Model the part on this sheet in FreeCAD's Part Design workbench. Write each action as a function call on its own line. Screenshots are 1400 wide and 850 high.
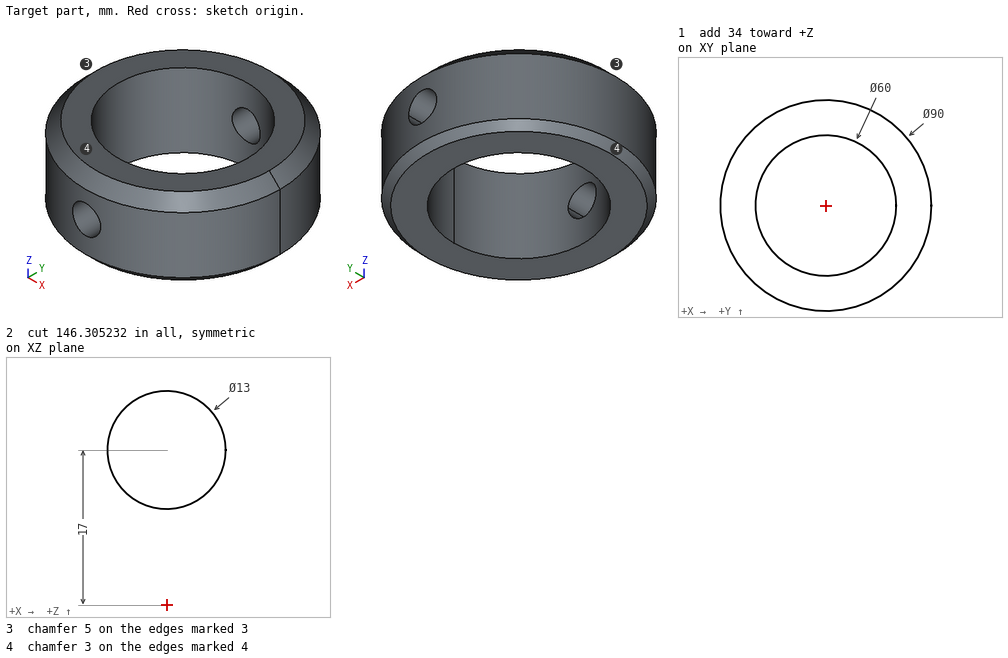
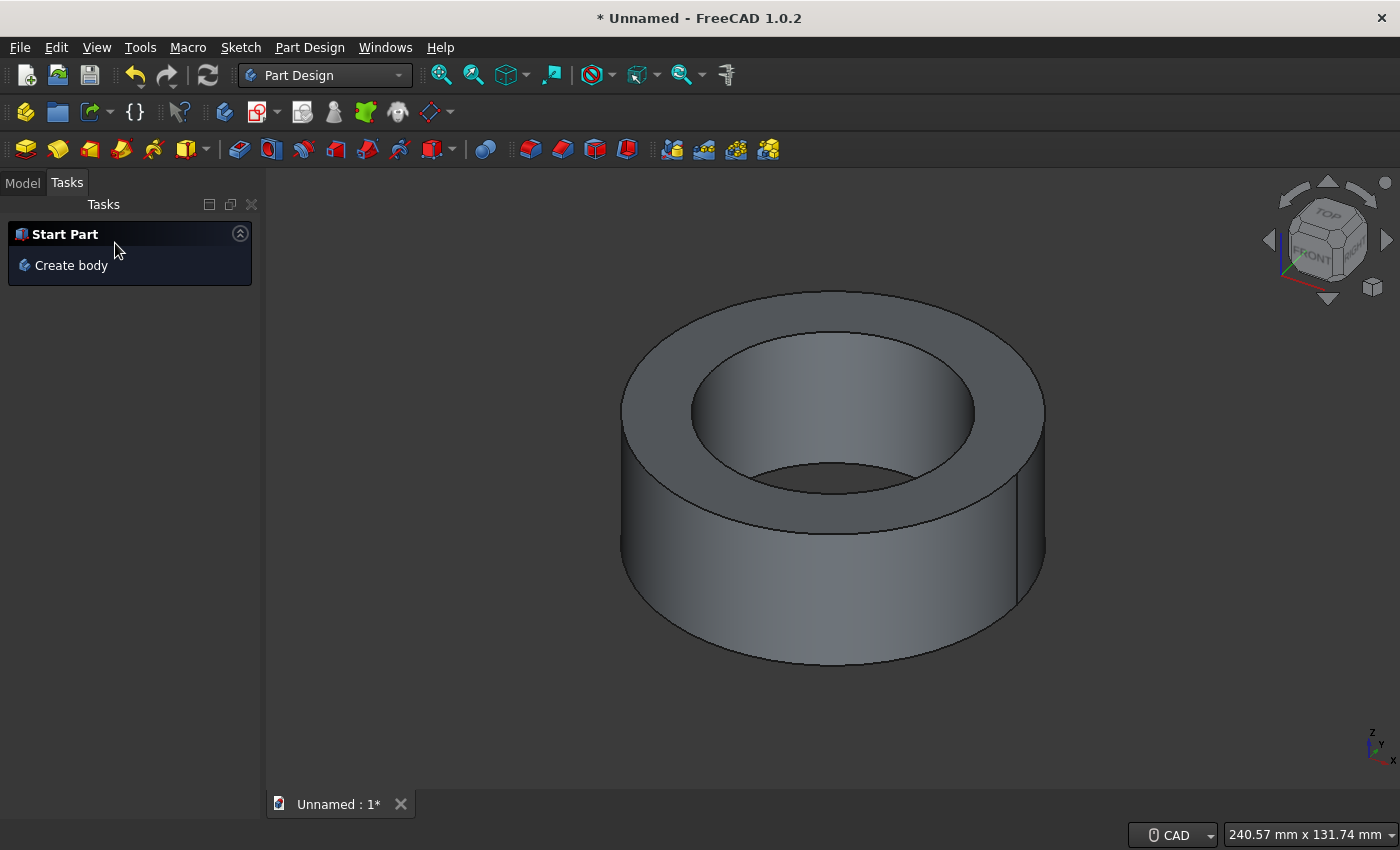
click(258, 112)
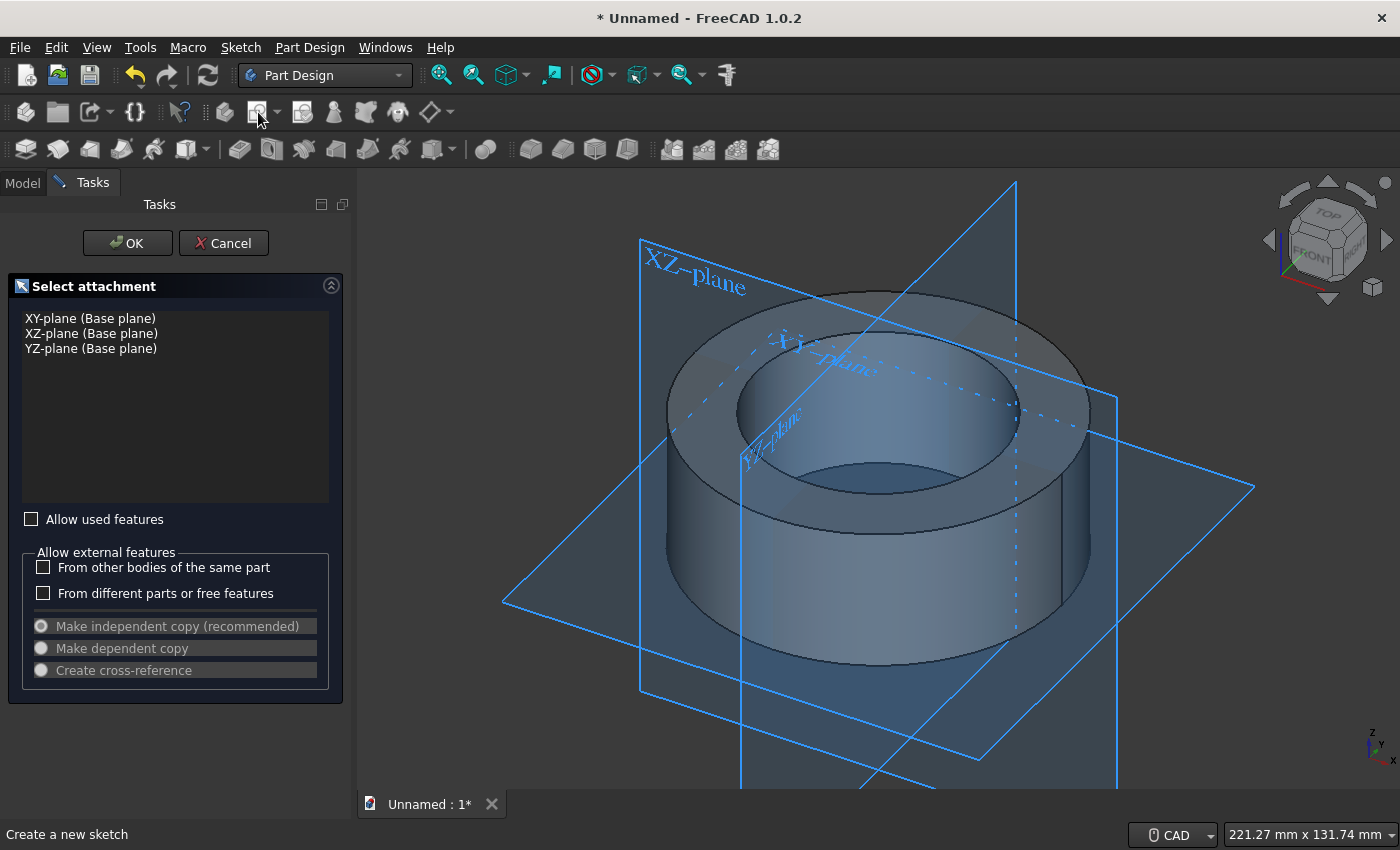
click(82, 334)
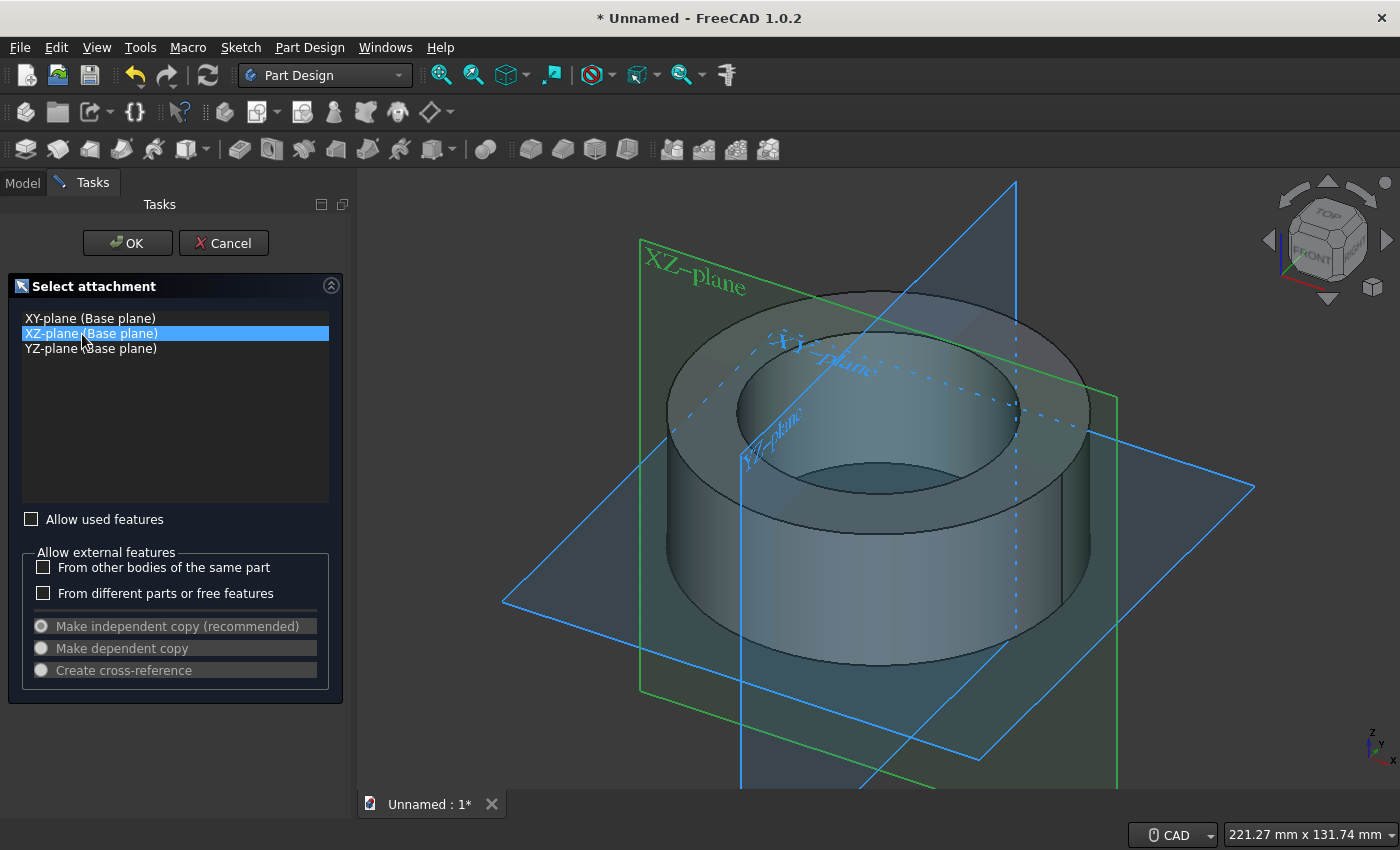
click(128, 243)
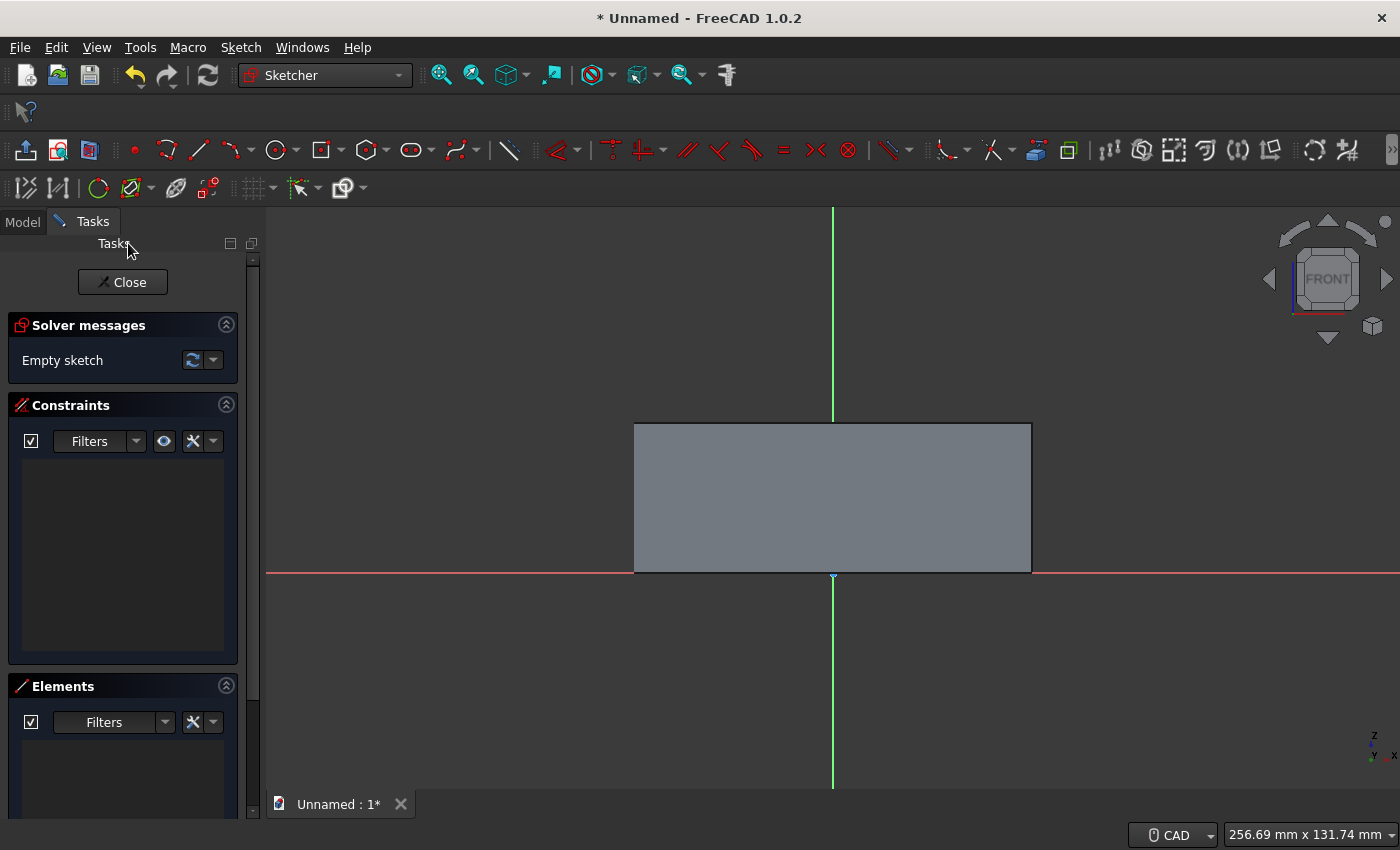
key(q)
key(s)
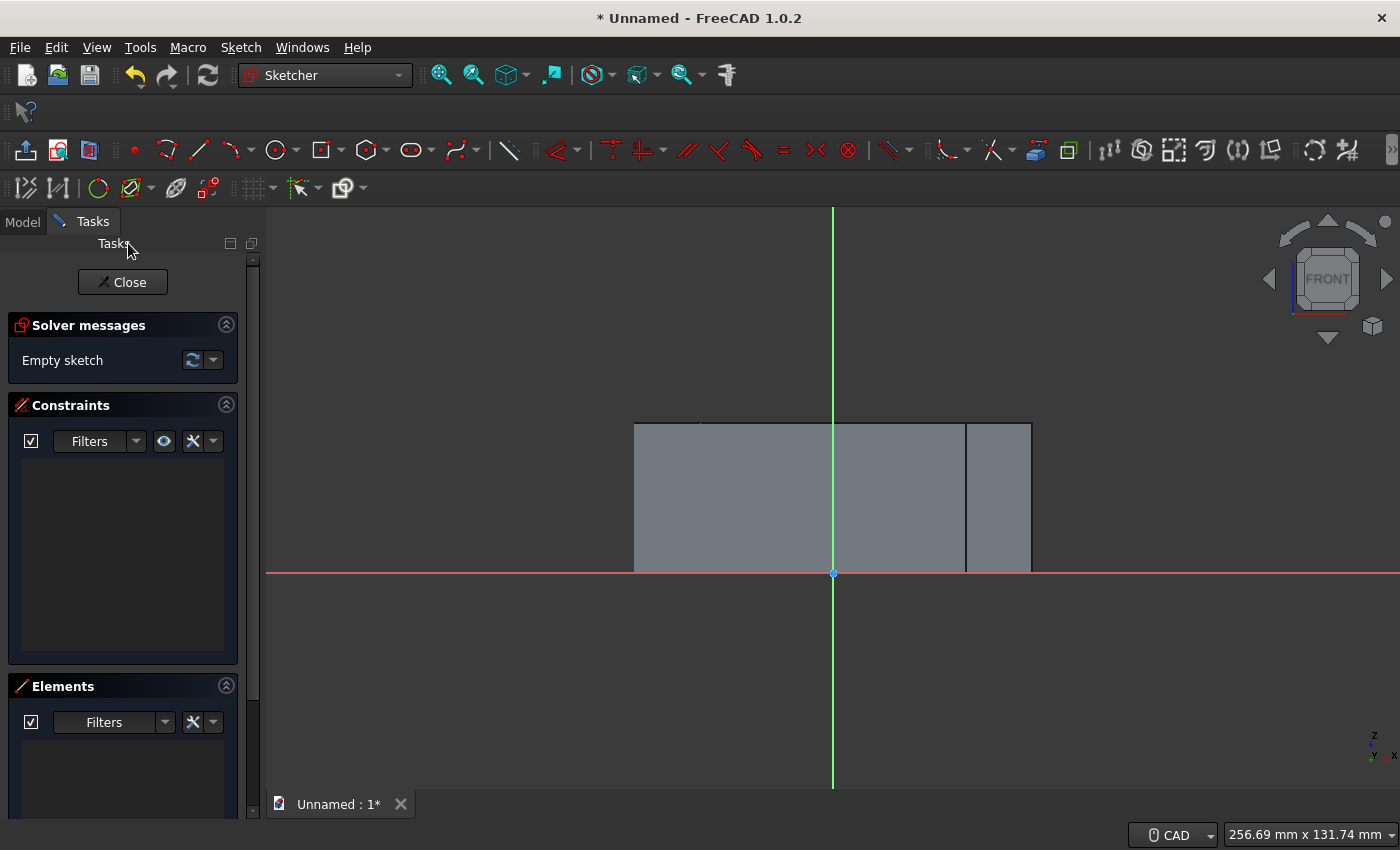
scroll(863, 531, up, 6)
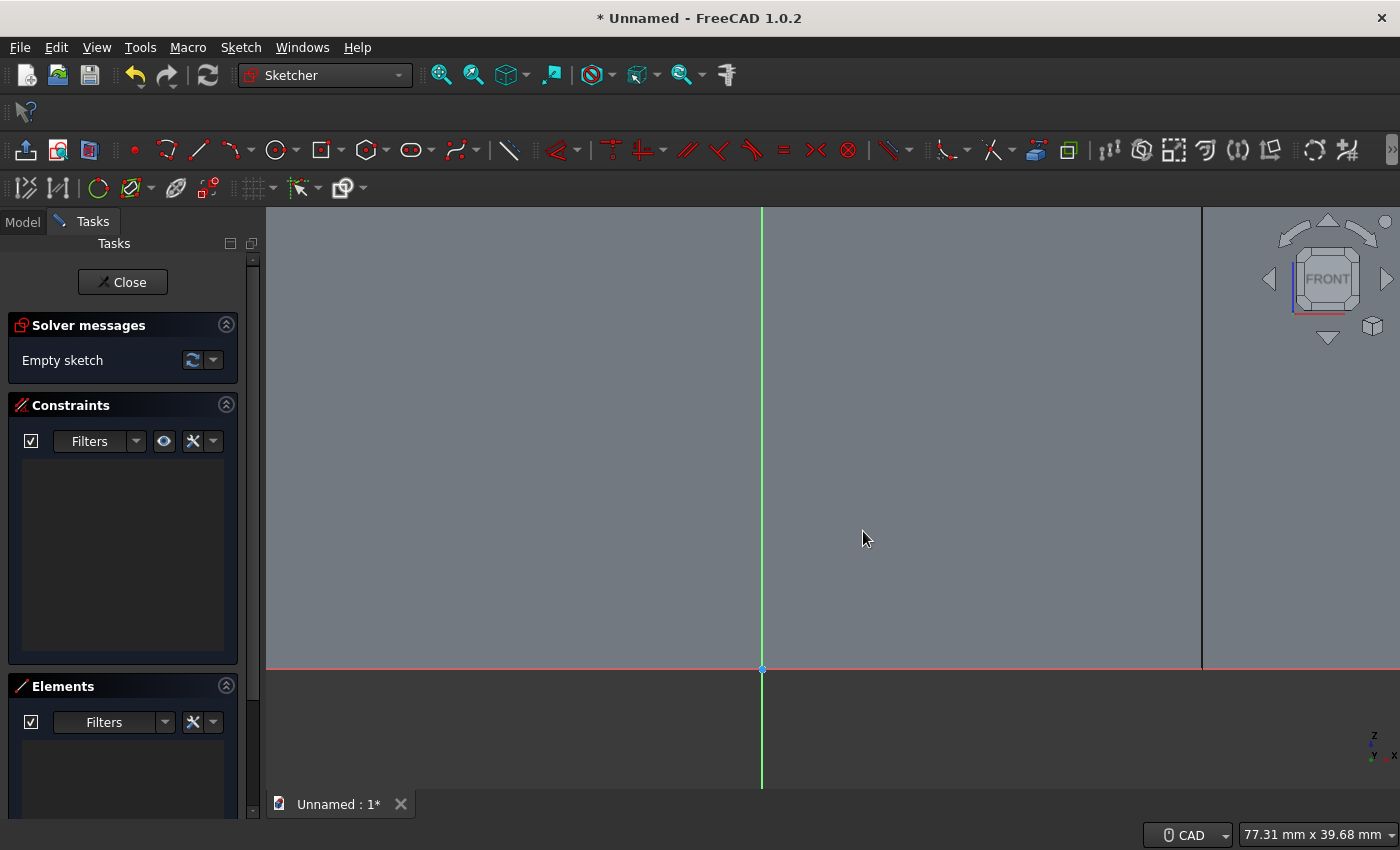
click(276, 150)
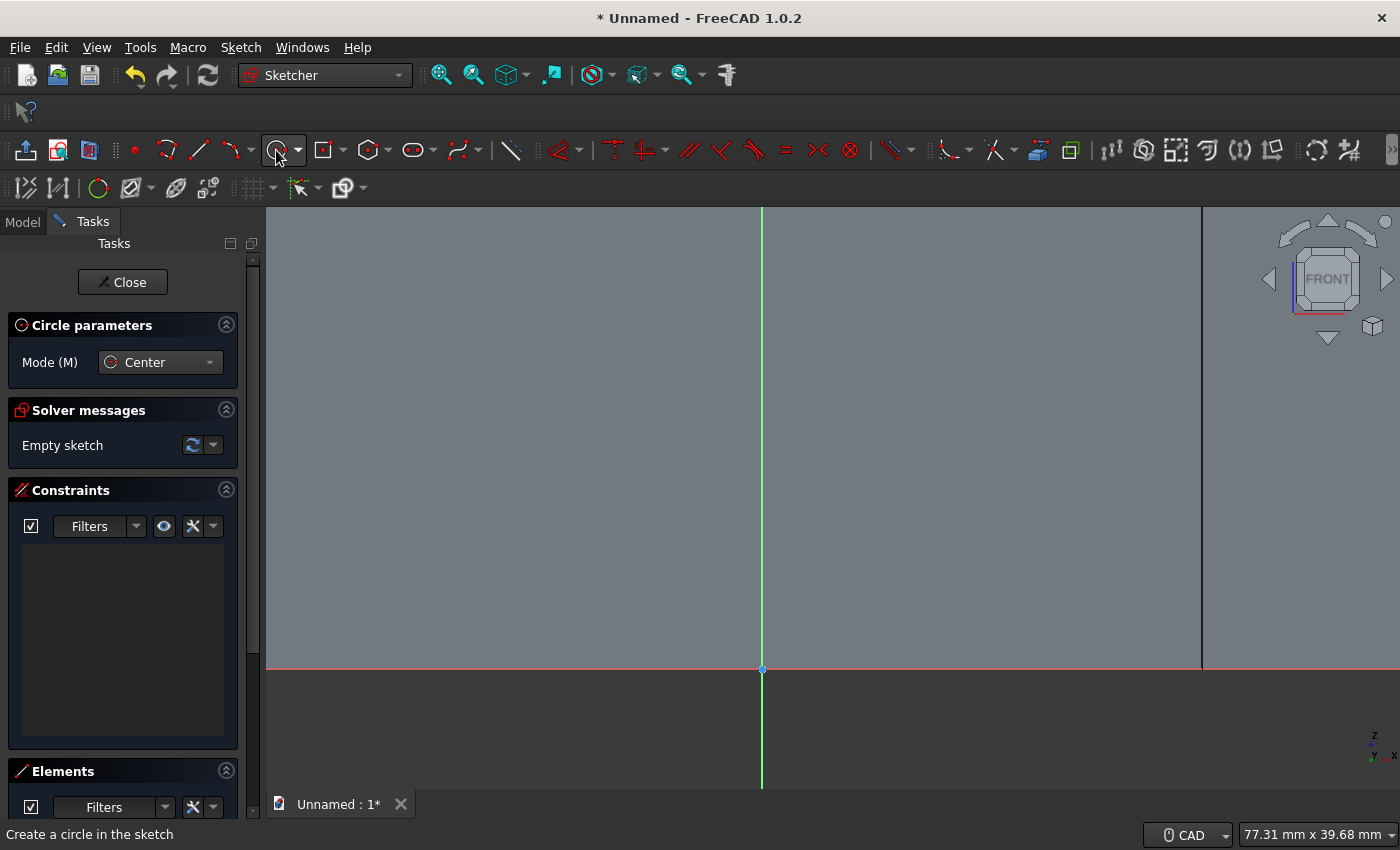
click(762, 420)
click(830, 353)
key(Escape)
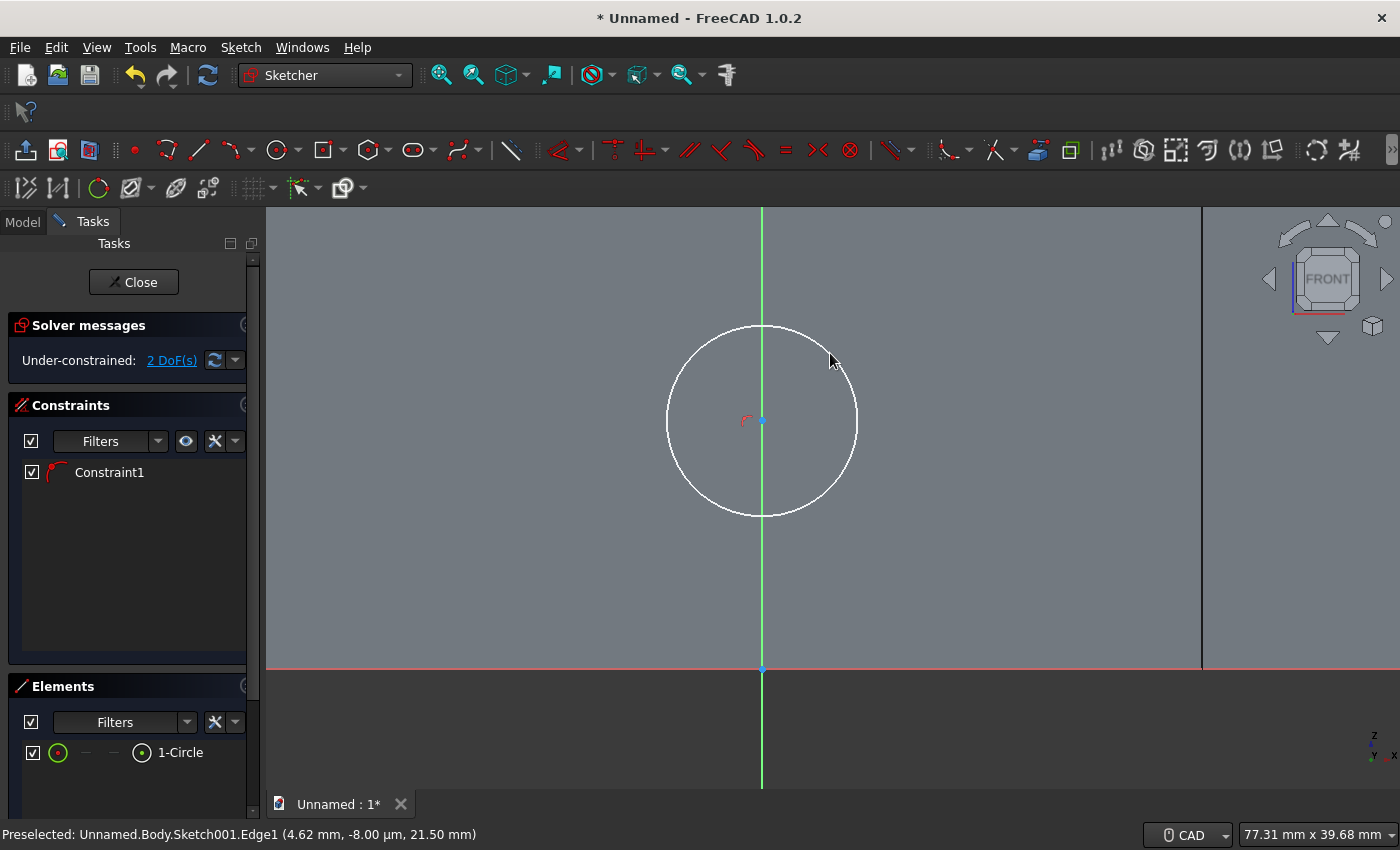
click(558, 150)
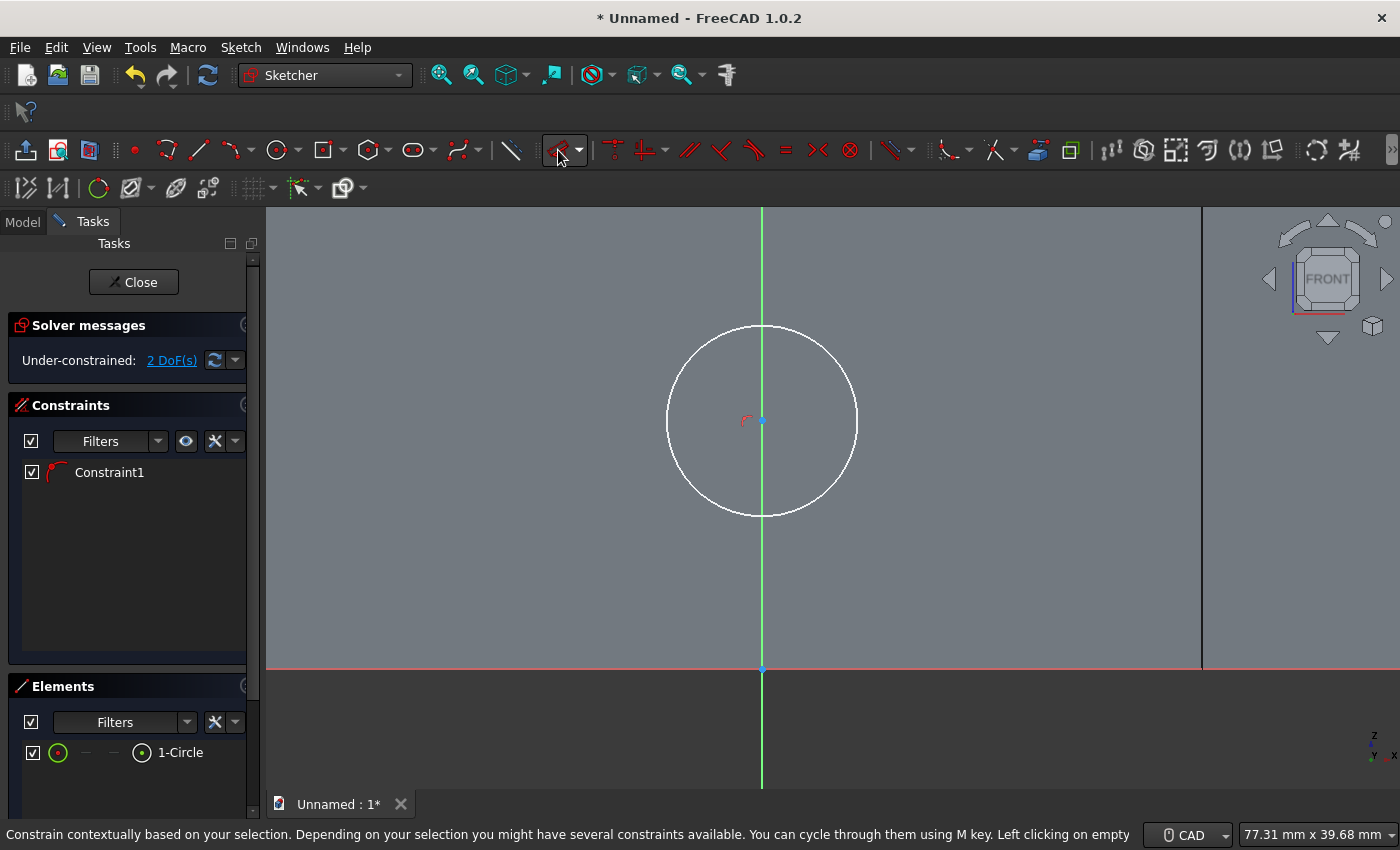
click(829, 353)
click(851, 330)